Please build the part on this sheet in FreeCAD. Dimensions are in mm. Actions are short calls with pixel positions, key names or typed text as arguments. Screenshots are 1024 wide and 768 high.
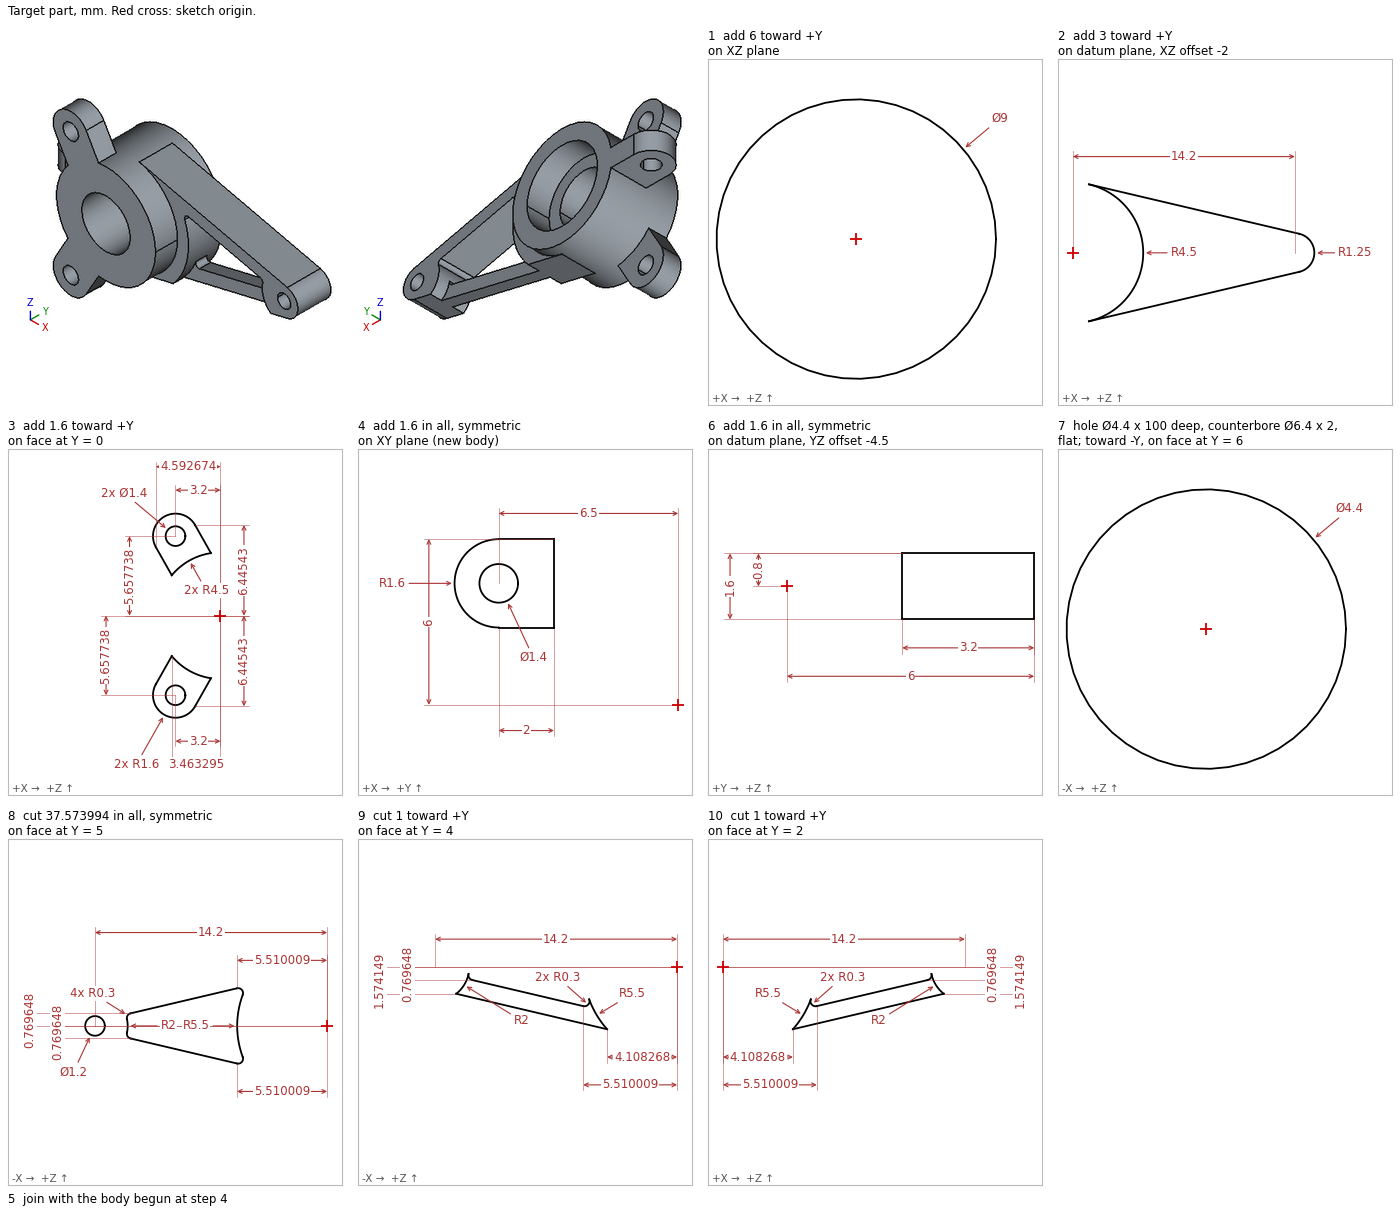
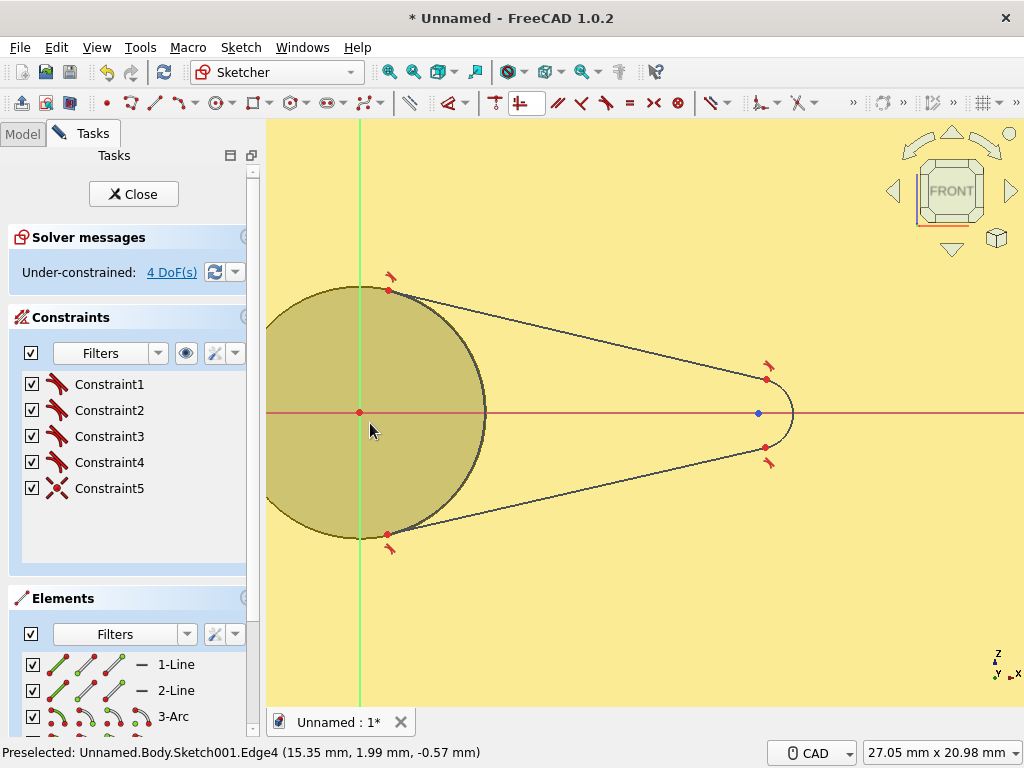
click(758, 414)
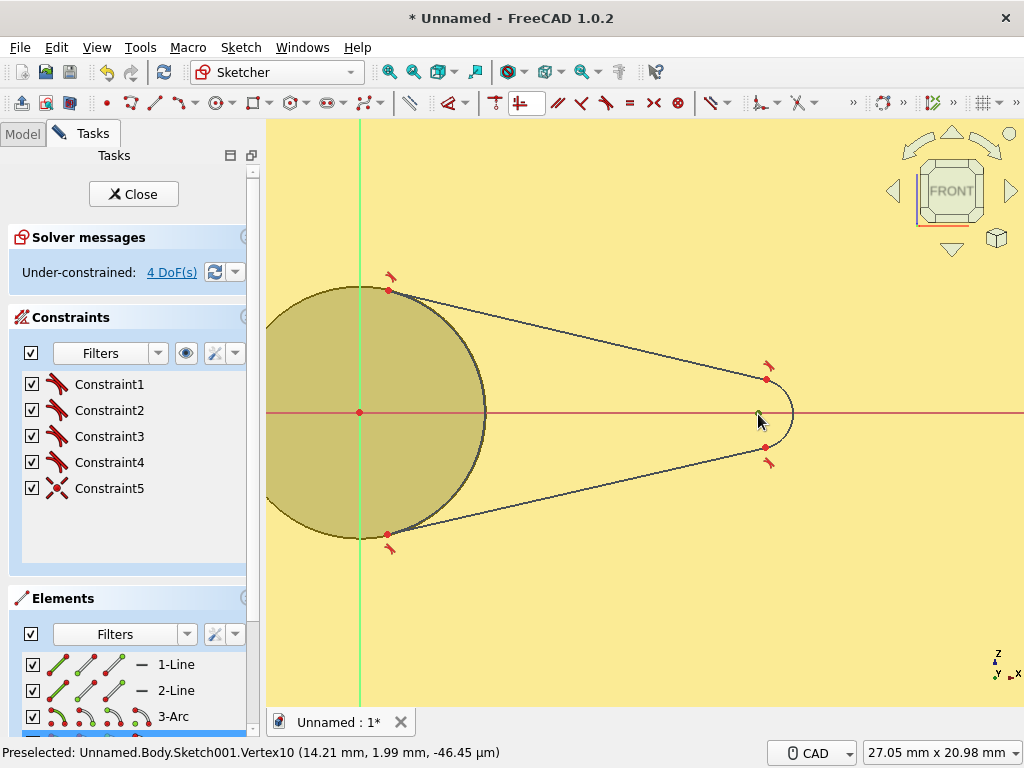
click(415, 413)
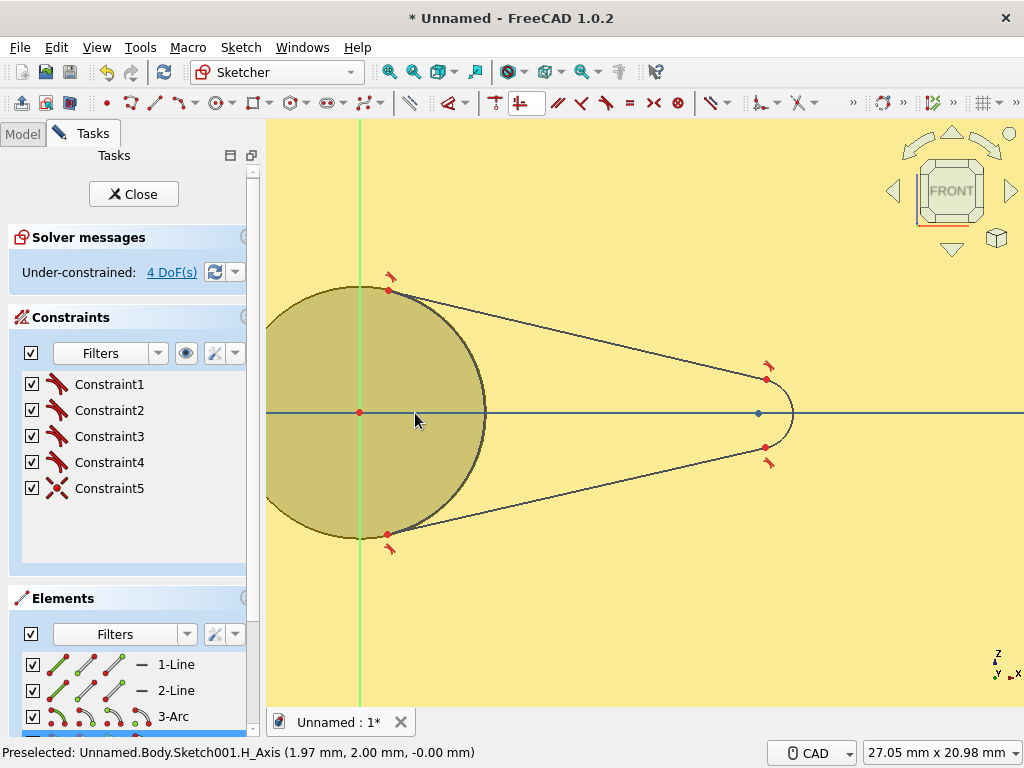
key(c)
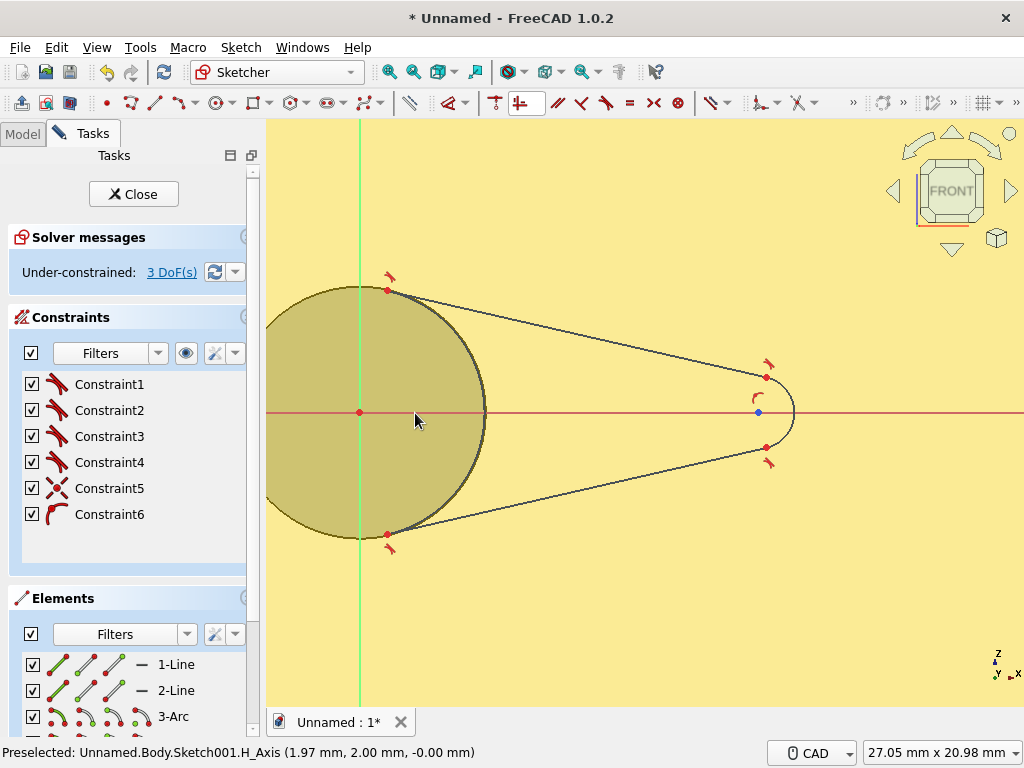
key(d)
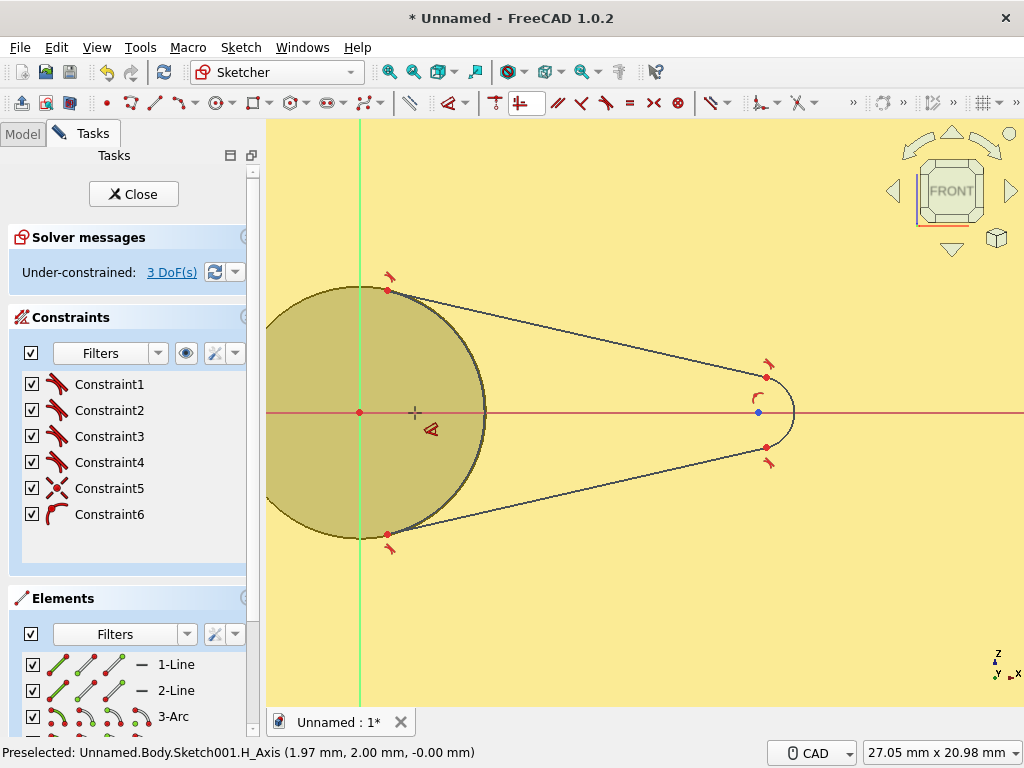
click(467, 477)
click(494, 493)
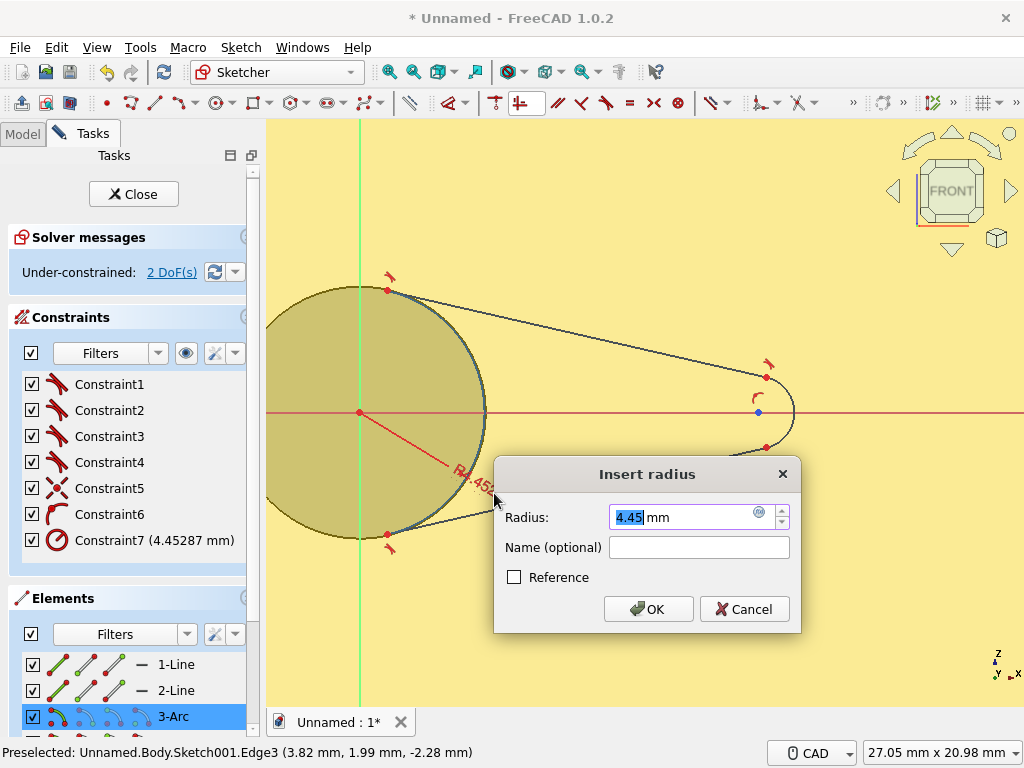
text(4.5)
key(Return)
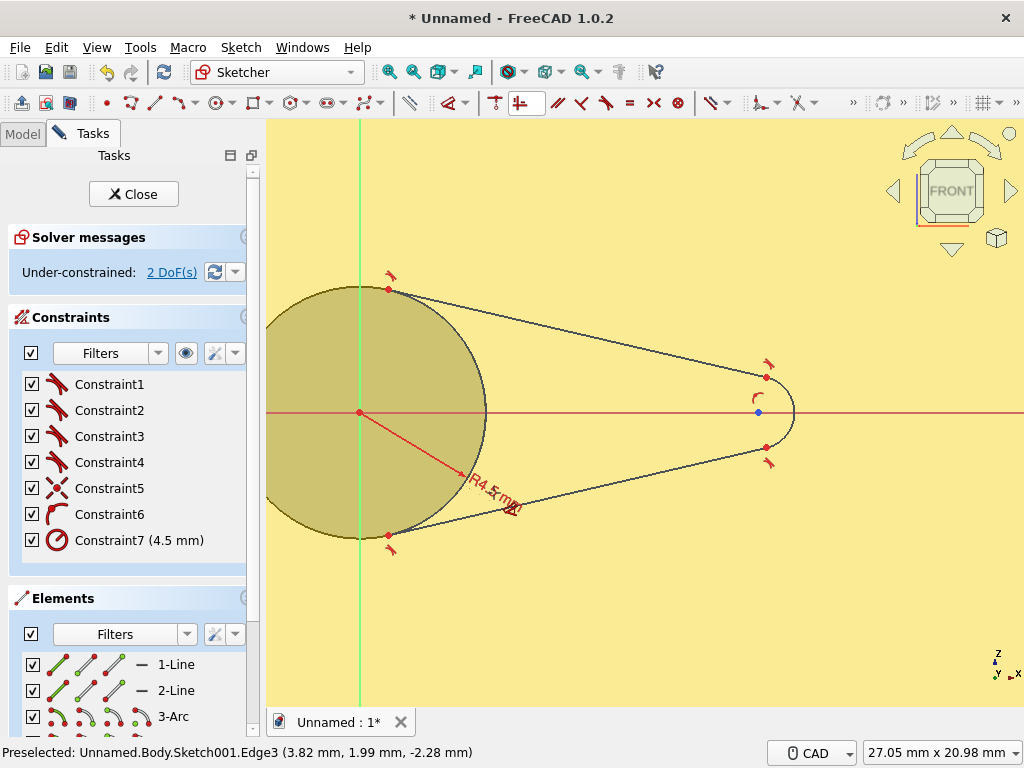
click(789, 431)
click(817, 447)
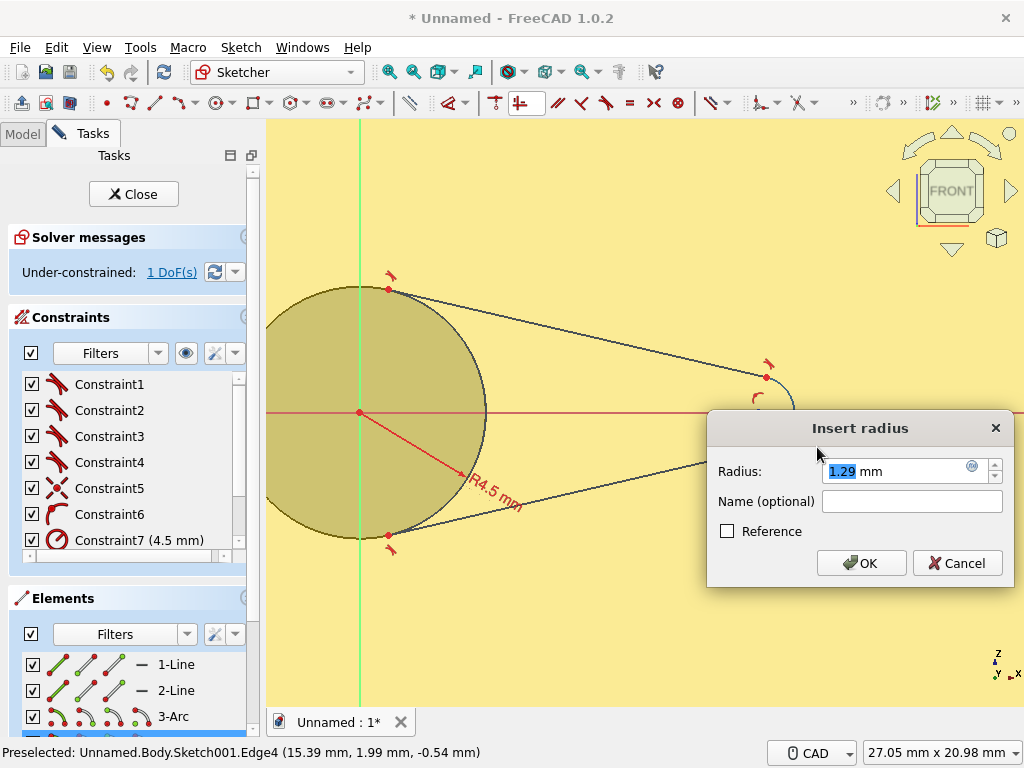
text(1.25)
key(Return)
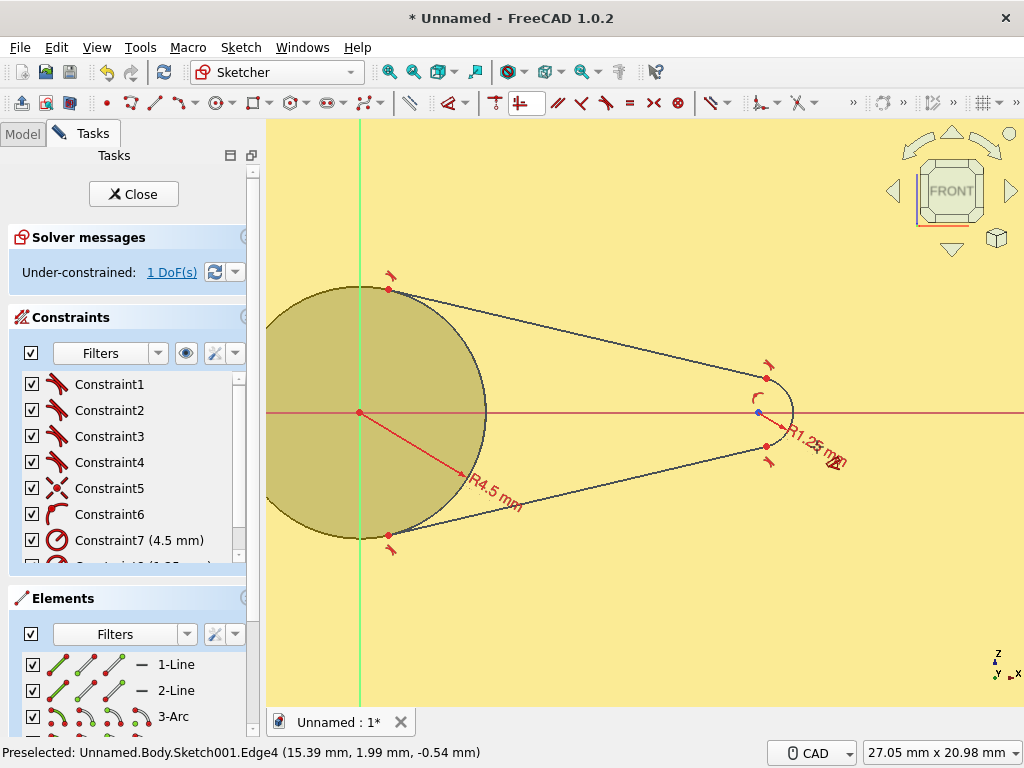
click(758, 413)
click(559, 447)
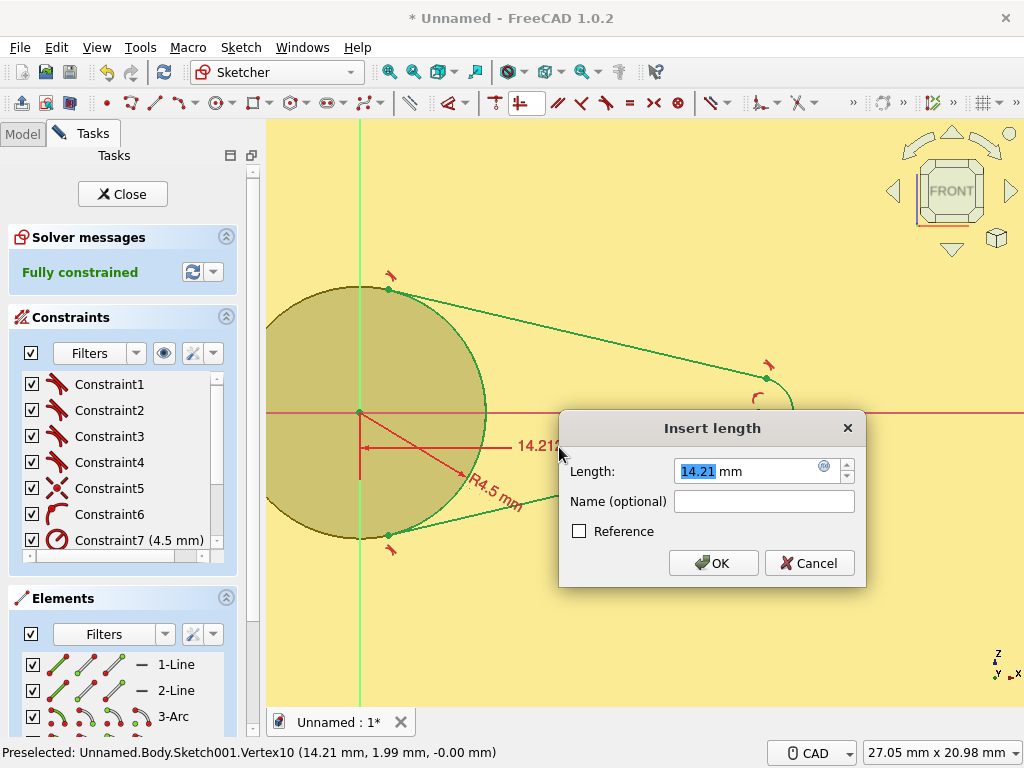
text(14.2)
key(Return)
key(Escape)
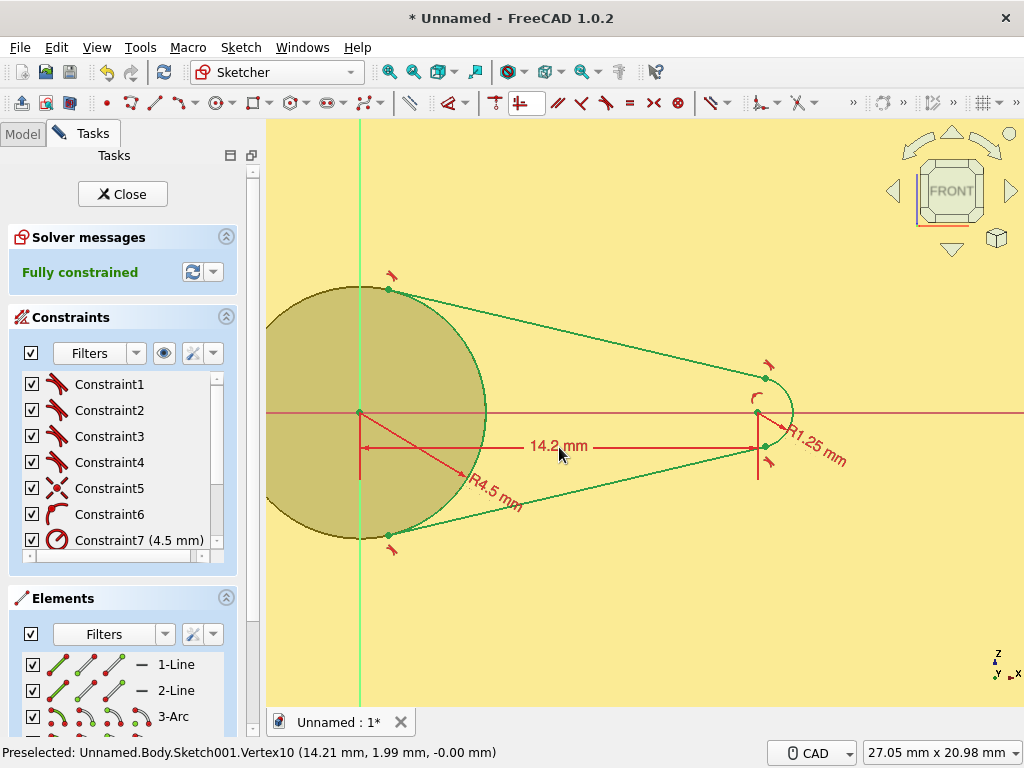
click(123, 194)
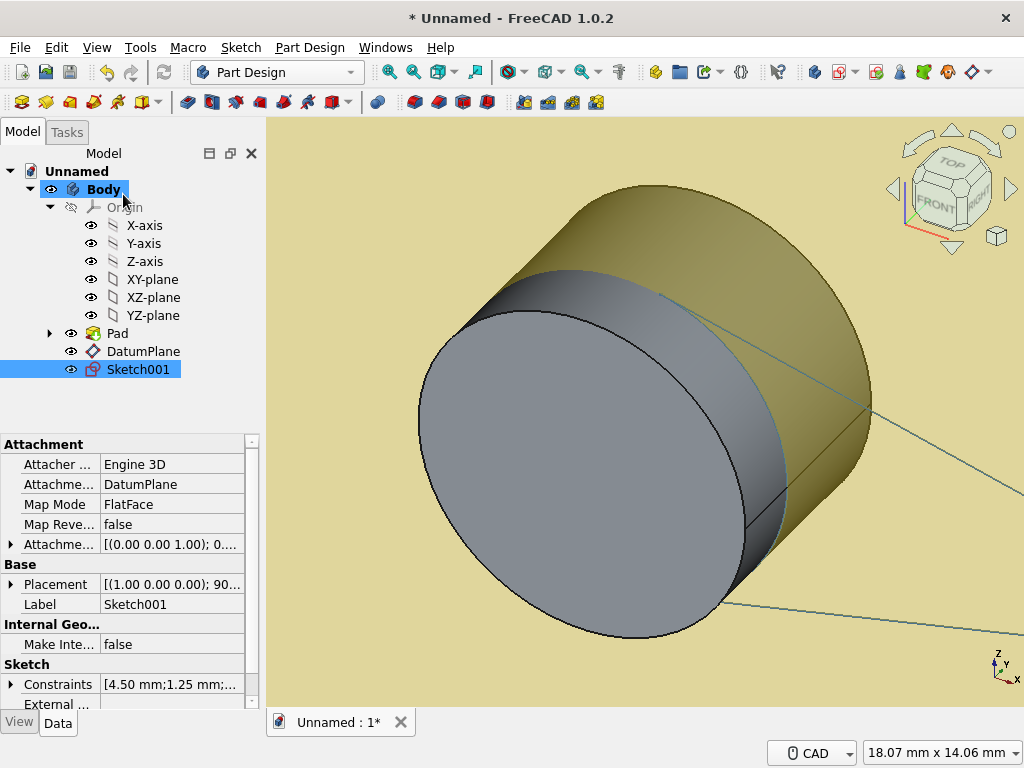
click(22, 102)